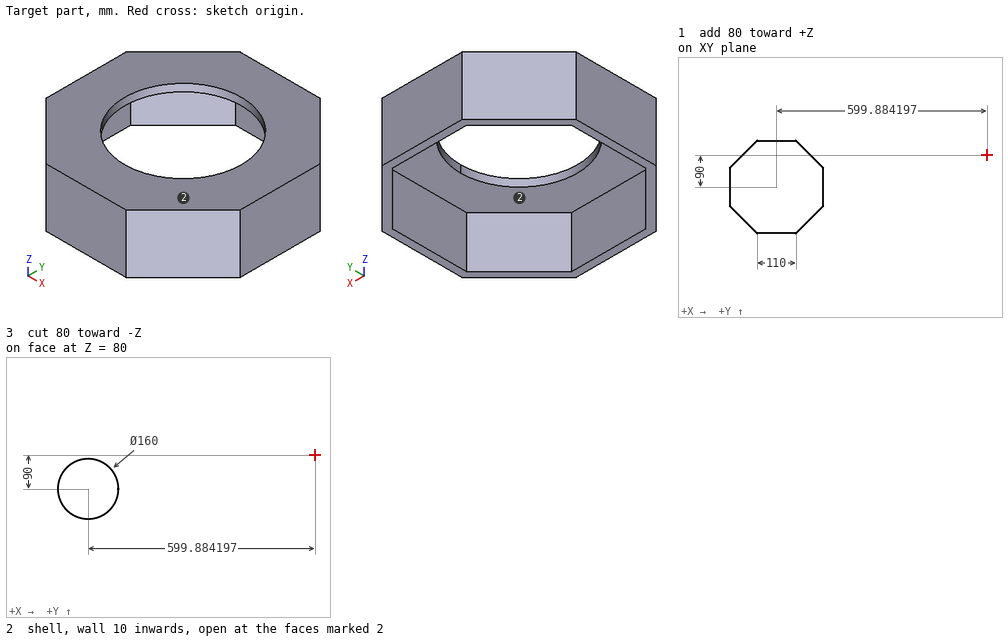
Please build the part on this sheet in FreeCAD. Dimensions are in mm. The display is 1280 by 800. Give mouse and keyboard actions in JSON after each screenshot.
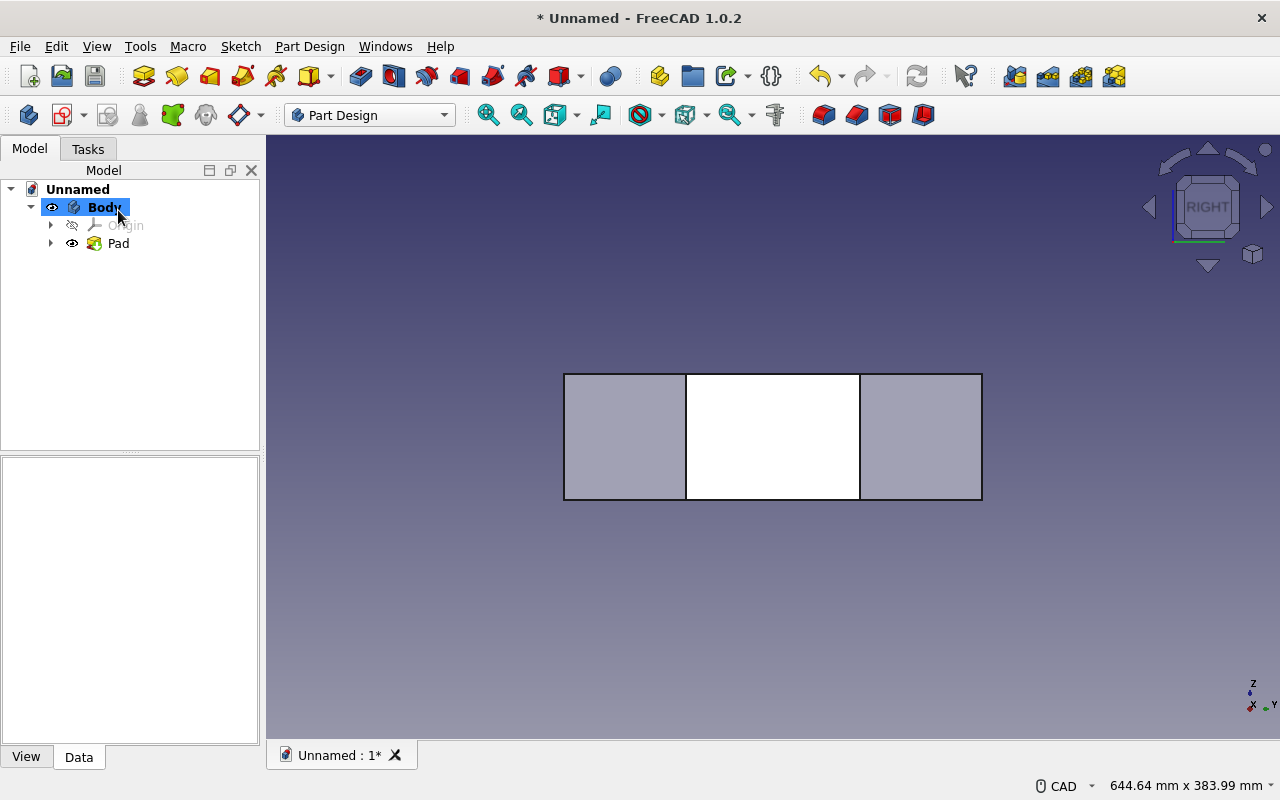
{"action": "key", "text": "v f"}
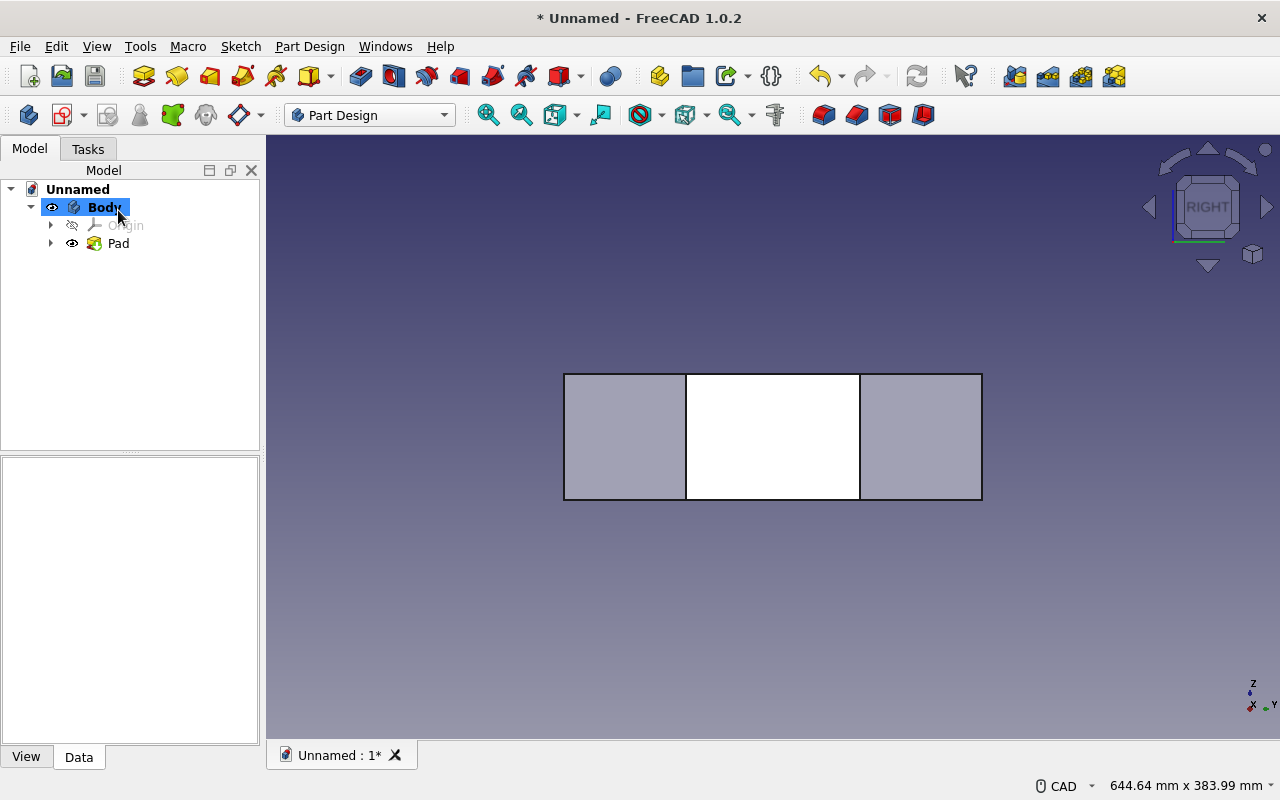
{"action": "key", "text": "5"}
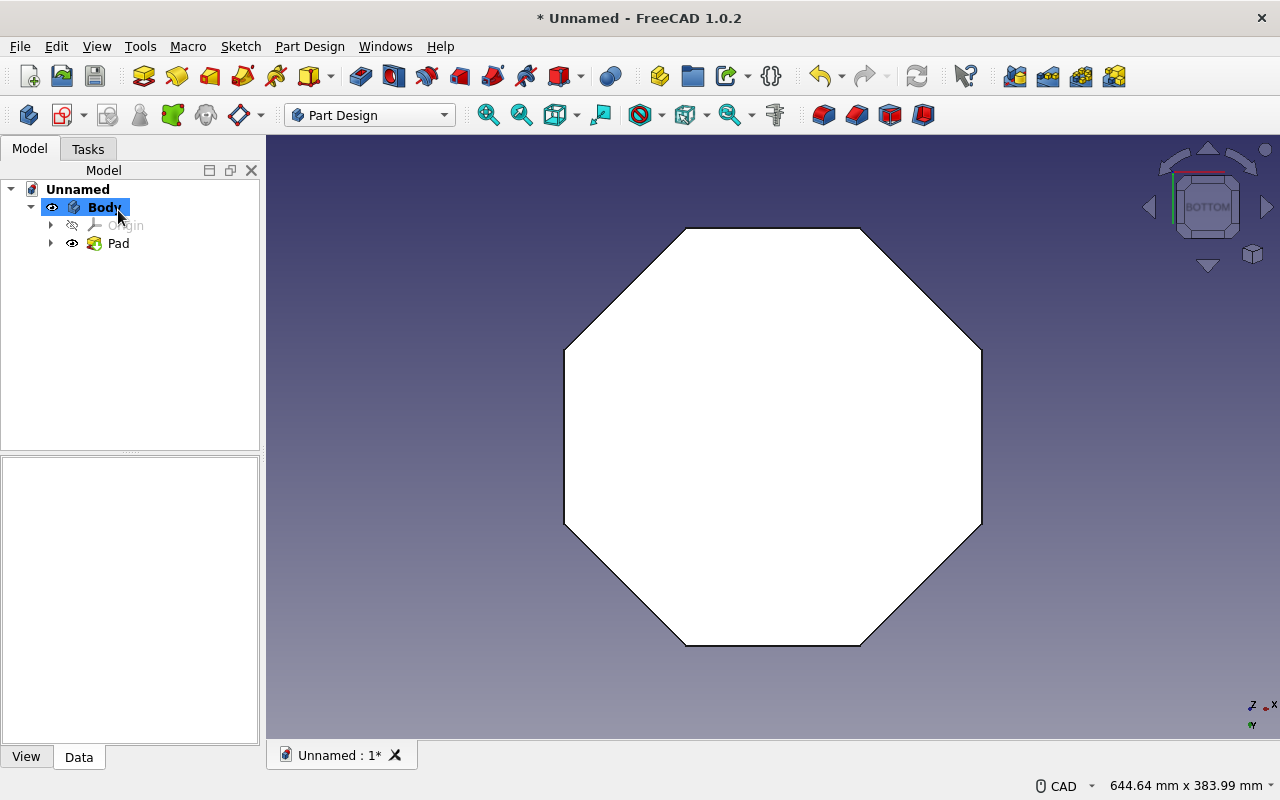
{"action": "left_click", "coordinate": [773, 436]}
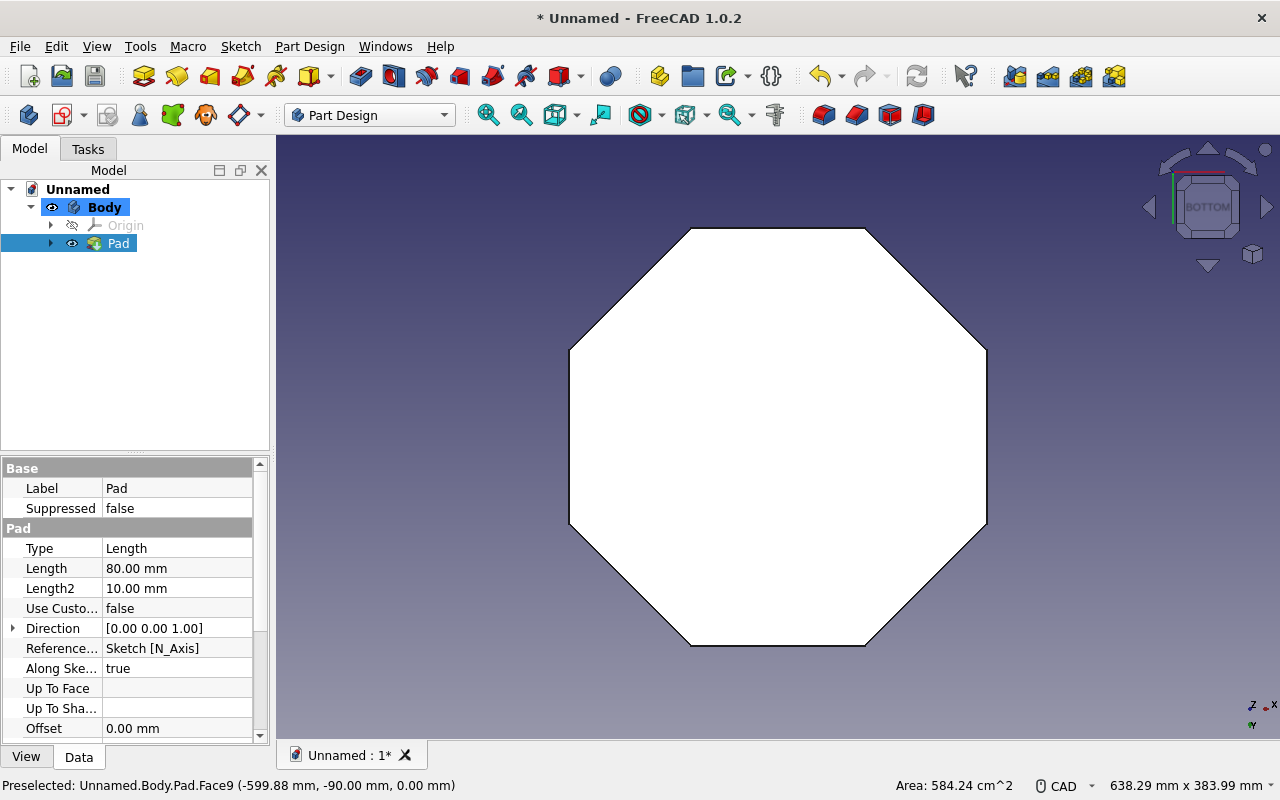
{"action": "left_click", "coordinate": [923, 116]}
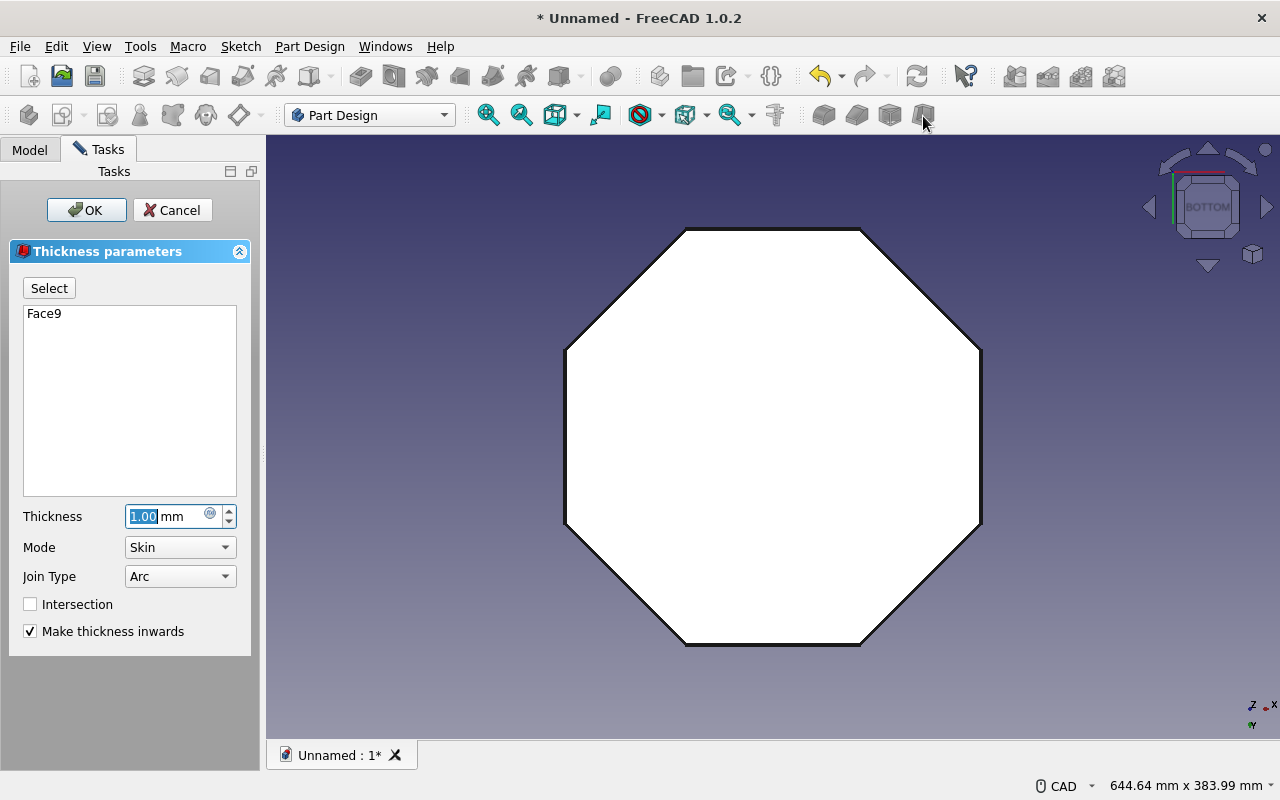
{"action": "type", "text": "10"}
{"action": "key", "text": "Tab"}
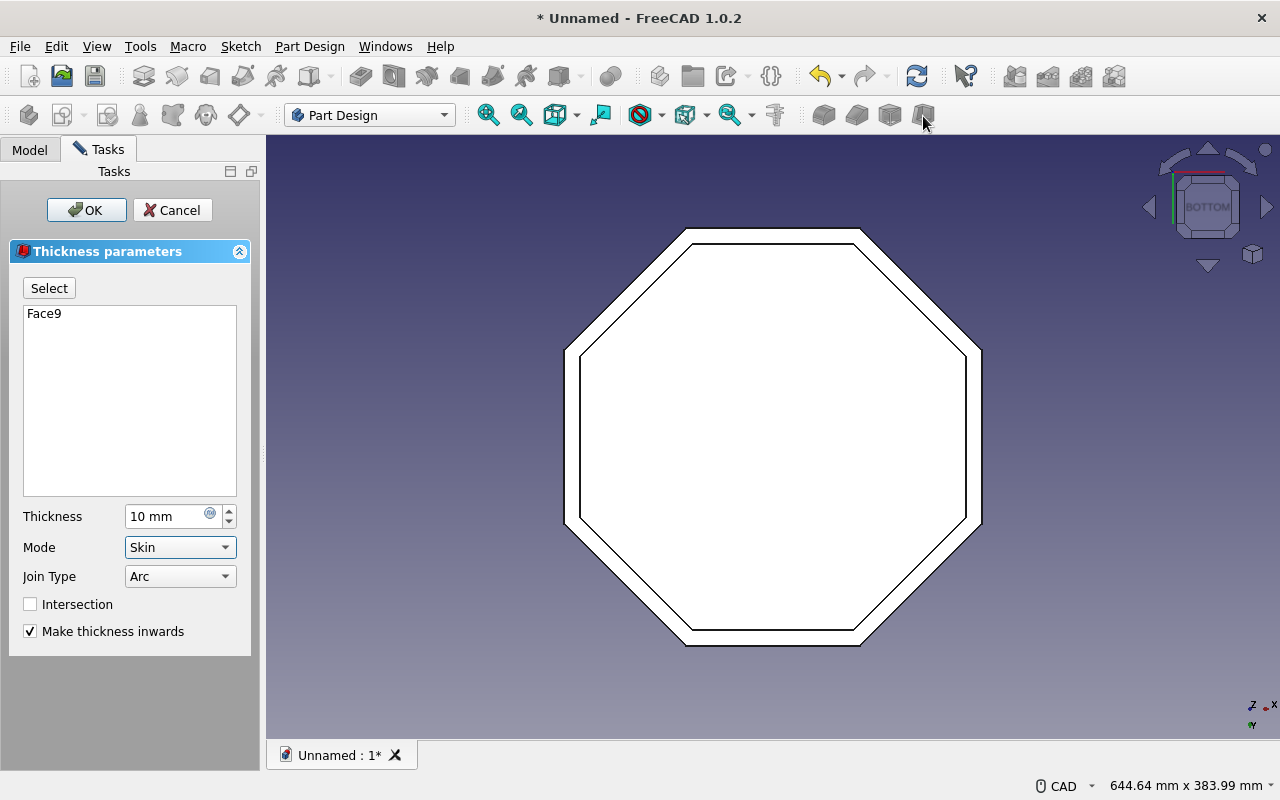
{"action": "left_click", "coordinate": [181, 576]}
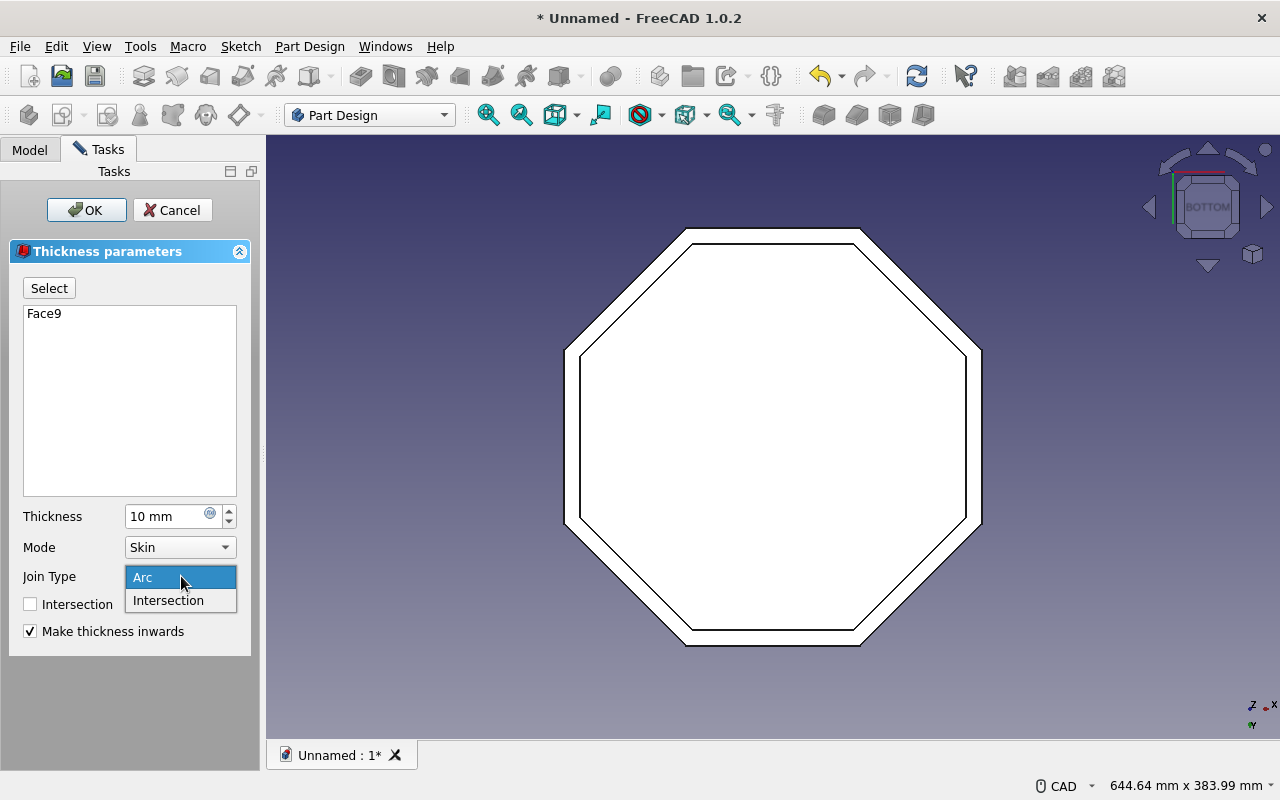
{"action": "left_click", "coordinate": [179, 600]}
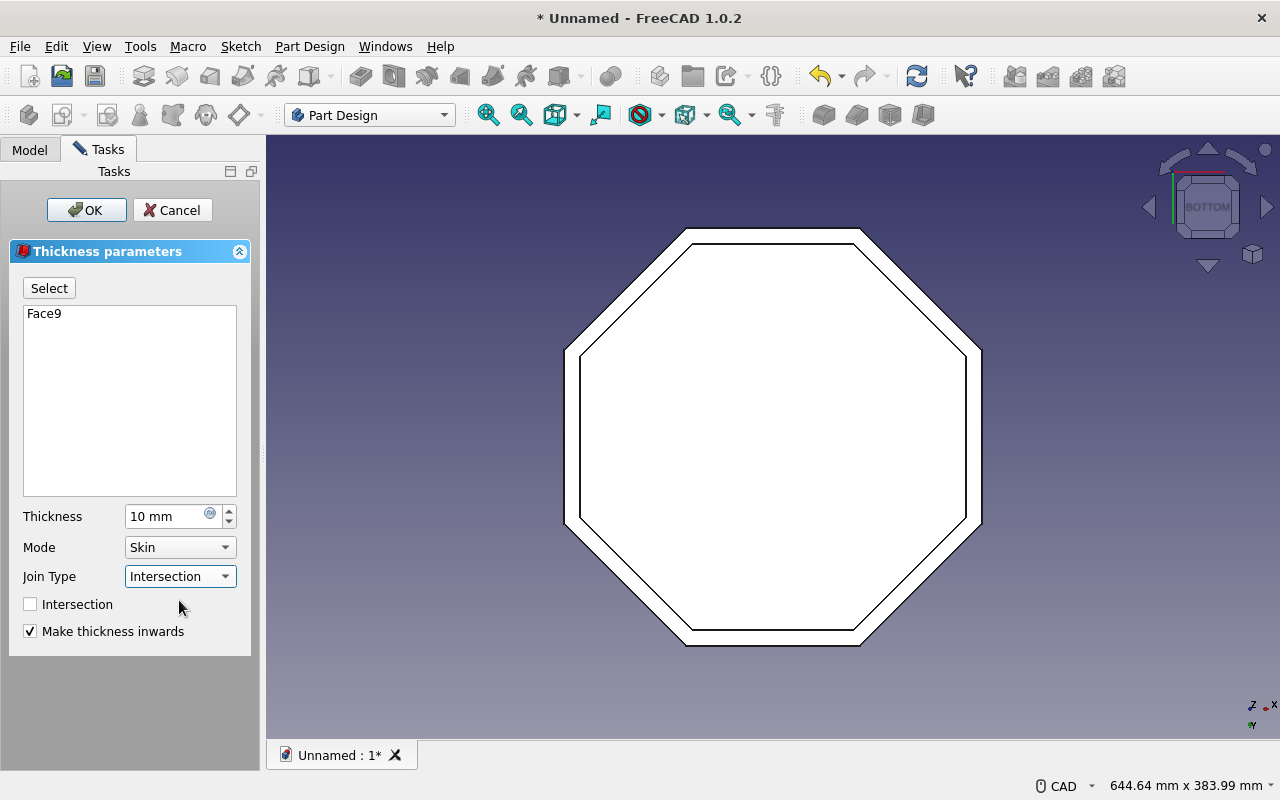
{"action": "left_click", "coordinate": [87, 210]}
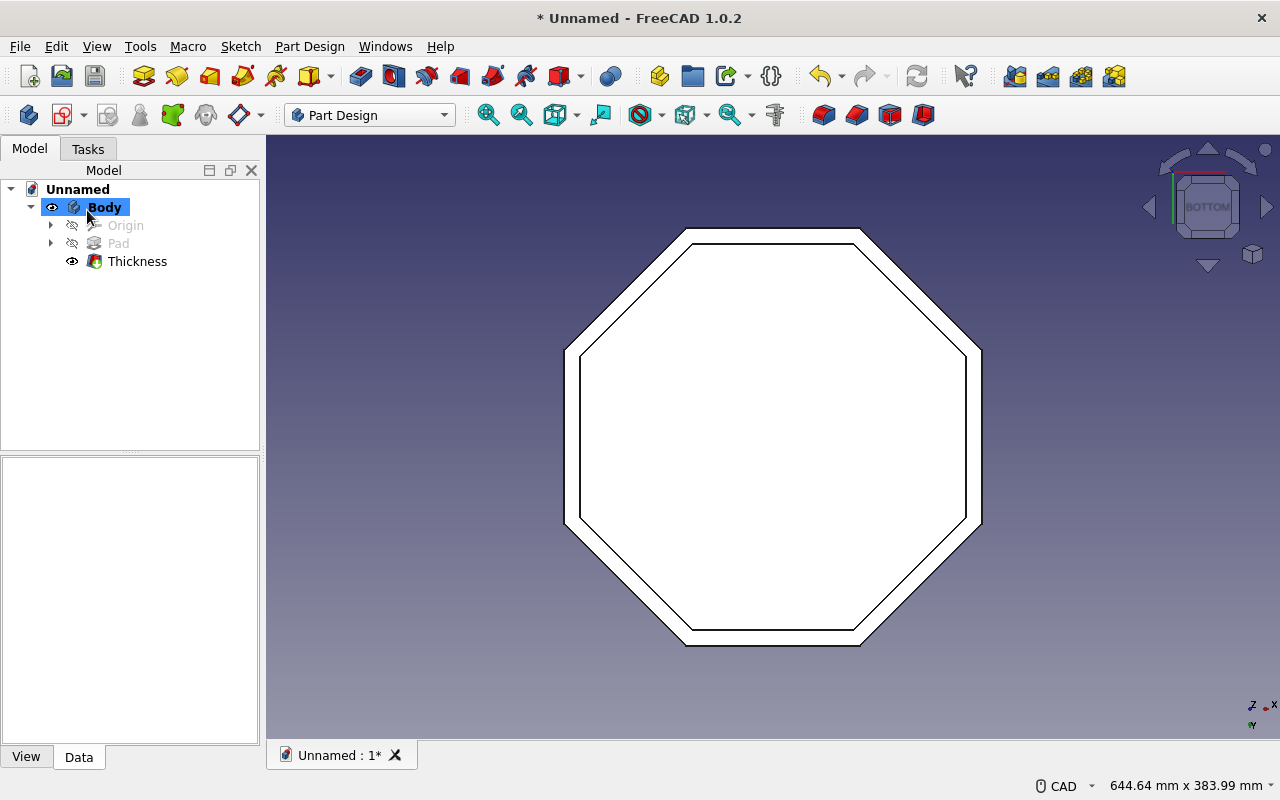
{"action": "key", "text": "0"}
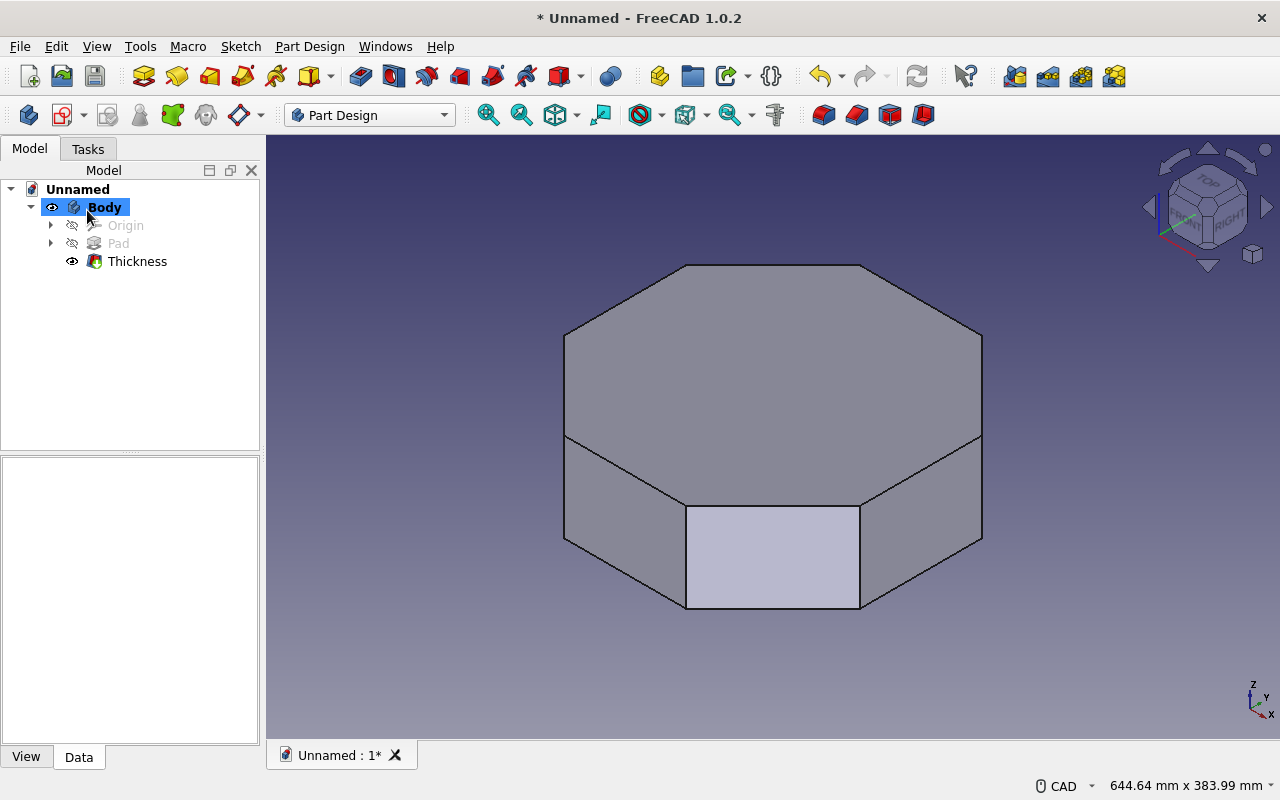
{"action": "left_click", "coordinate": [773, 385]}